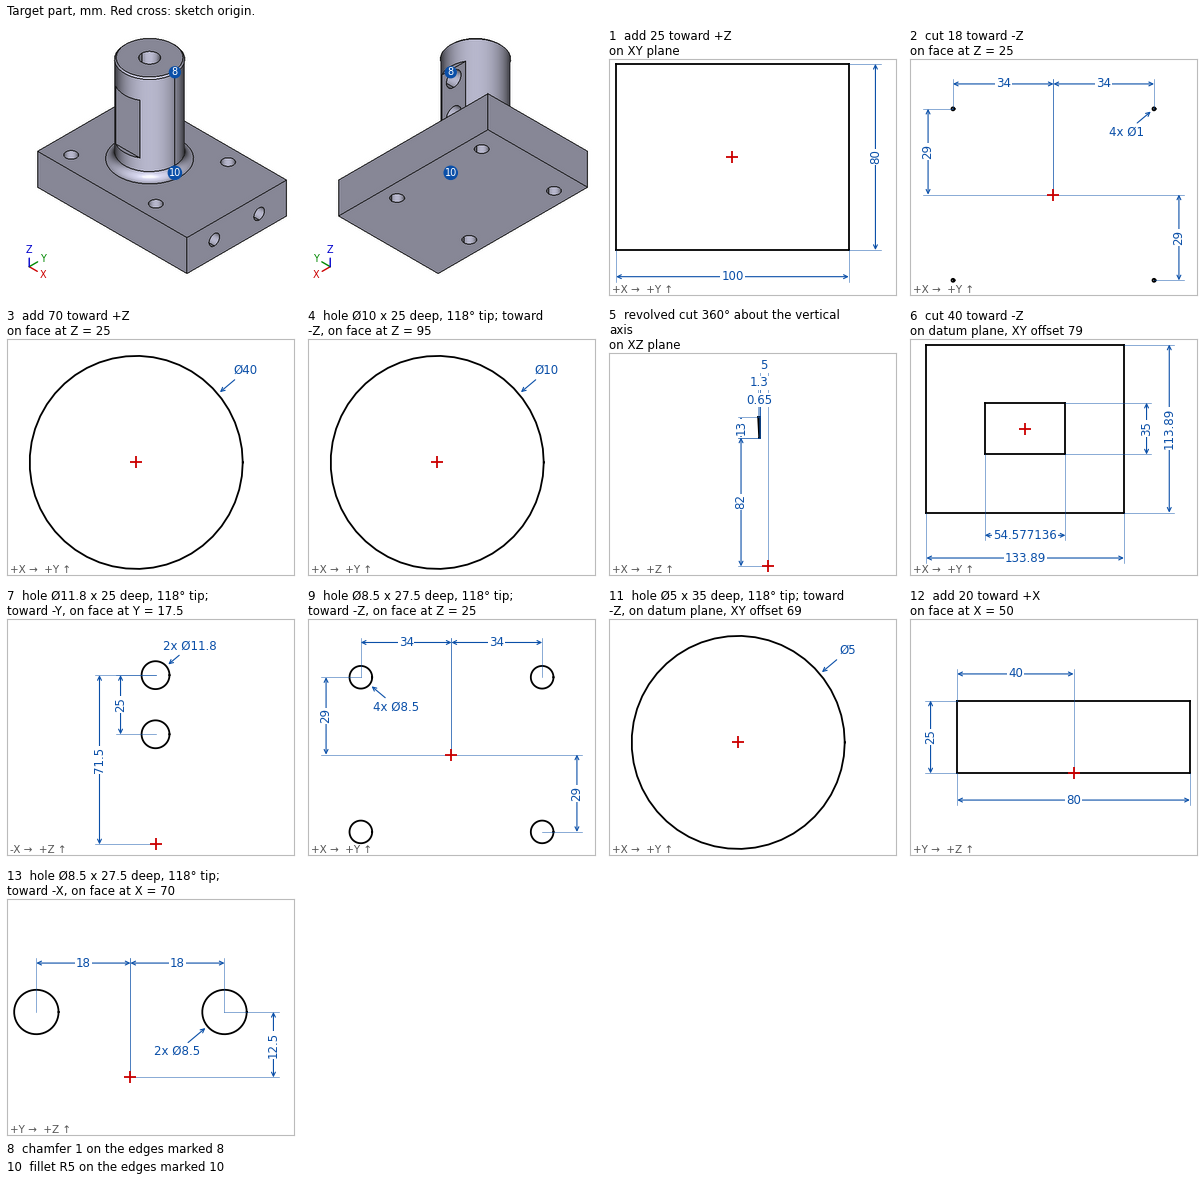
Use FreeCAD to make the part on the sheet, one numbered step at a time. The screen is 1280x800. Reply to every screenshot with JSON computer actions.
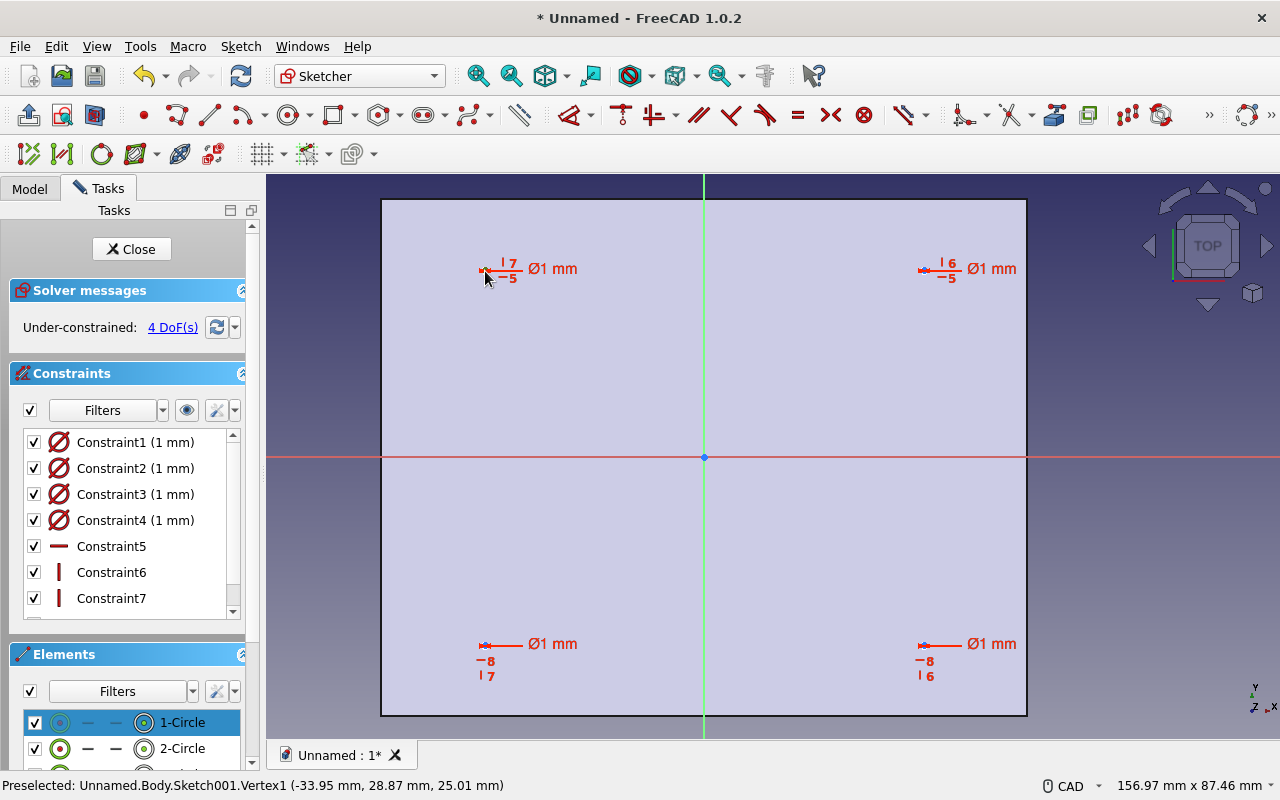
{"action": "key", "text": "l"}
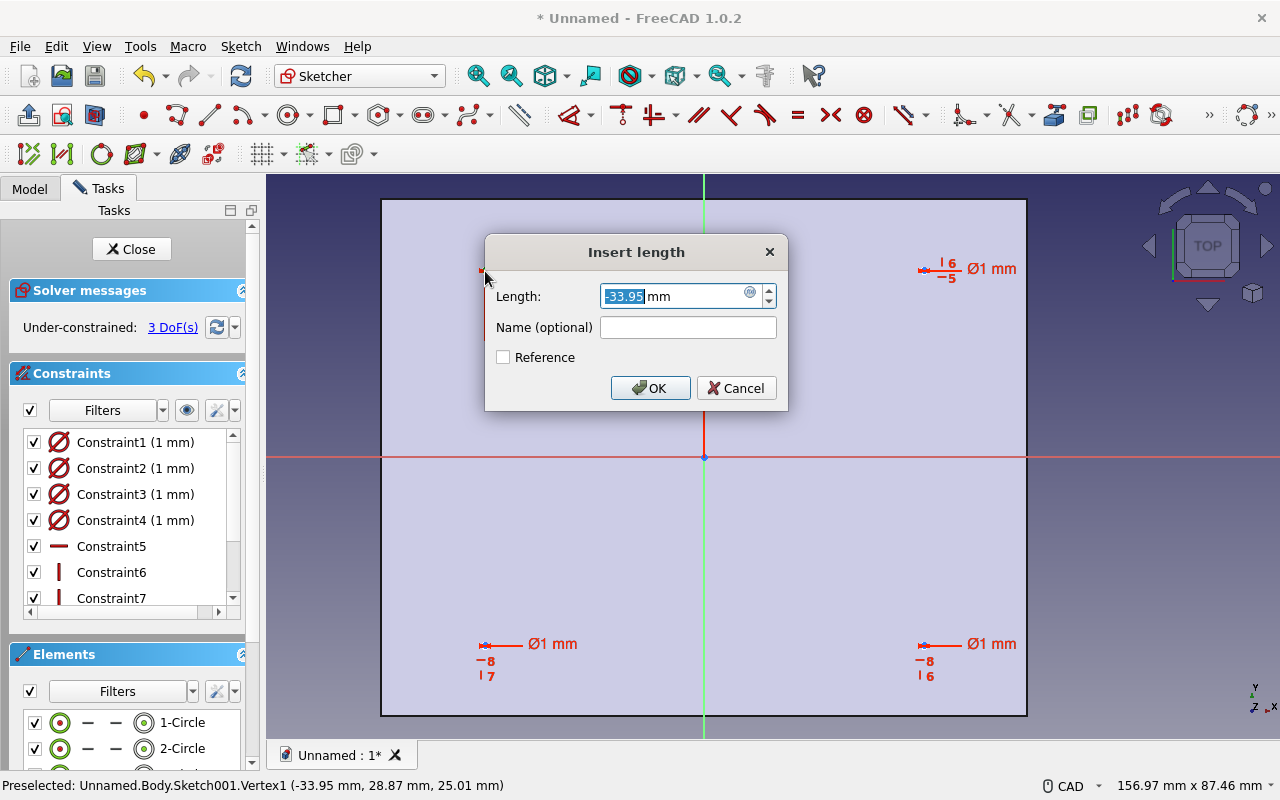
{"action": "type", "text": "-34"}
{"action": "key", "text": "Return"}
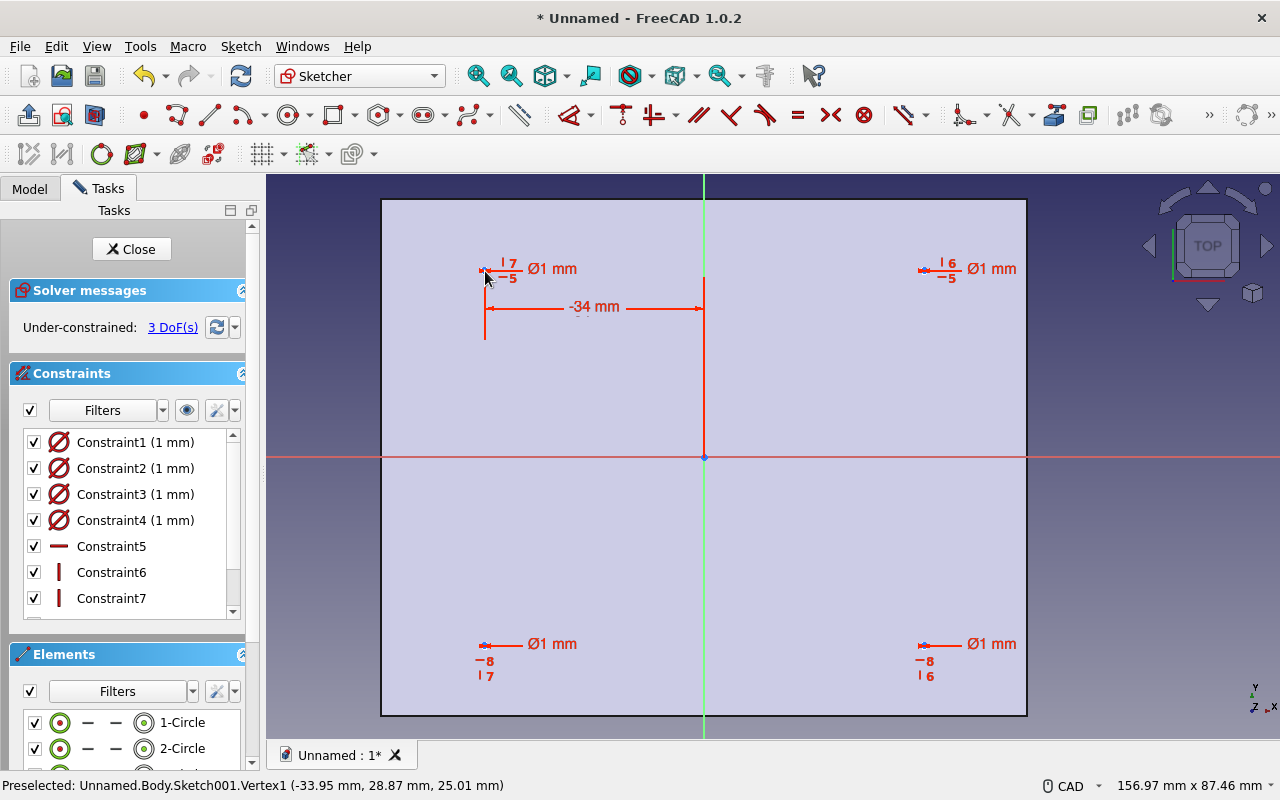
{"action": "left_click", "coordinate": [485, 271]}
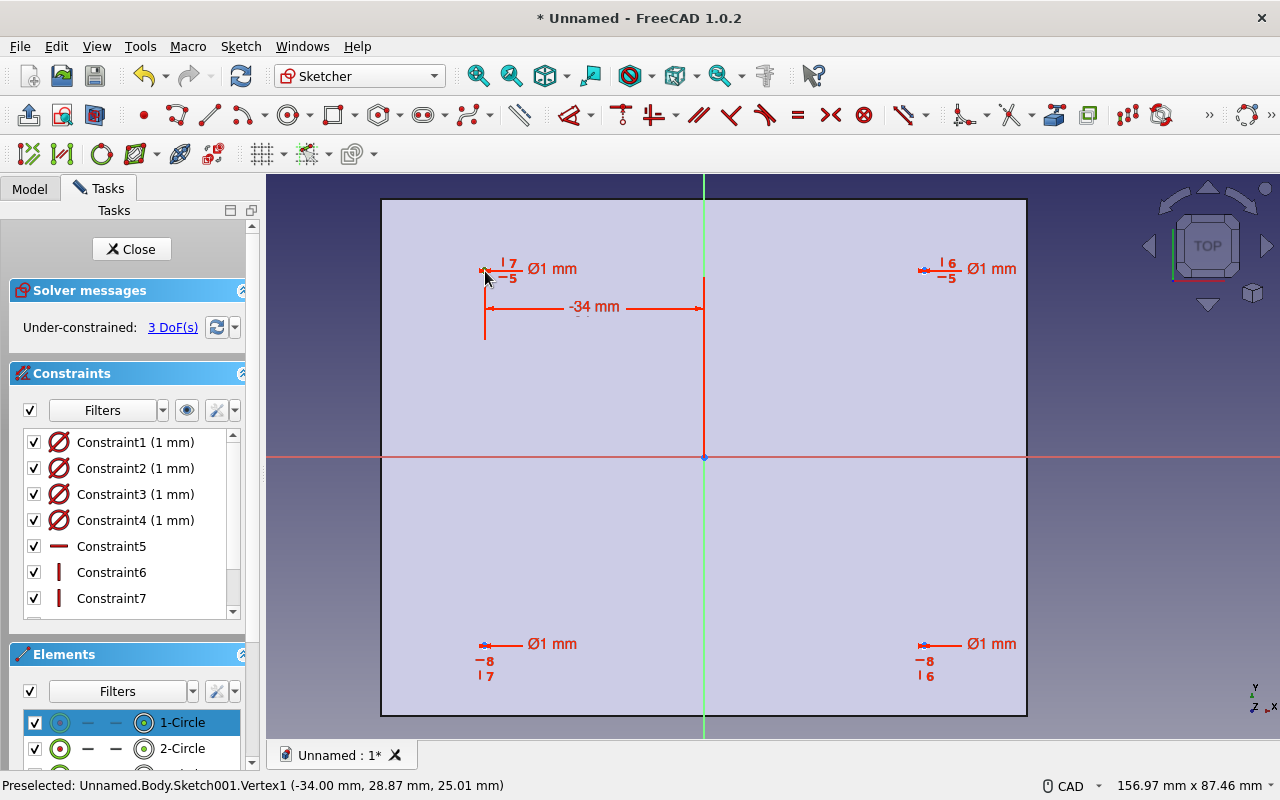
{"action": "key", "text": "i"}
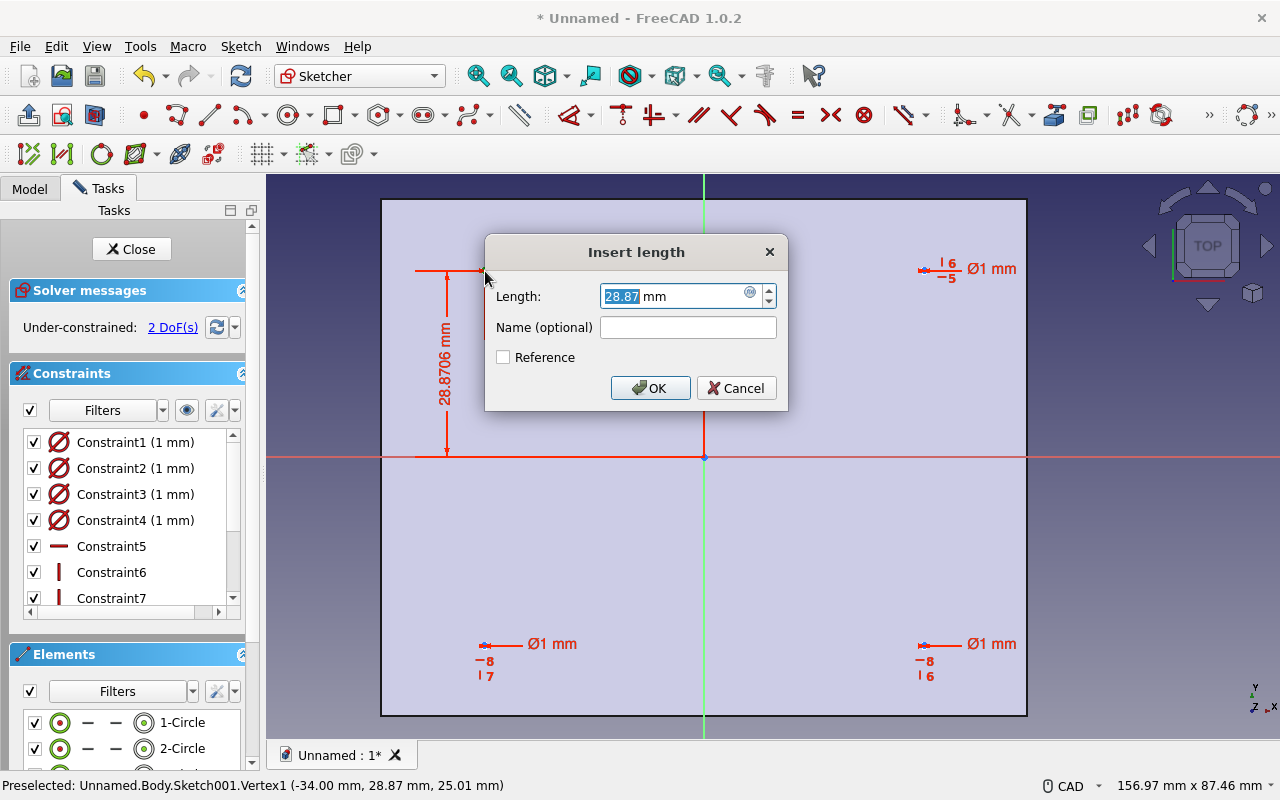
{"action": "type", "text": "29"}
{"action": "key", "text": "Return"}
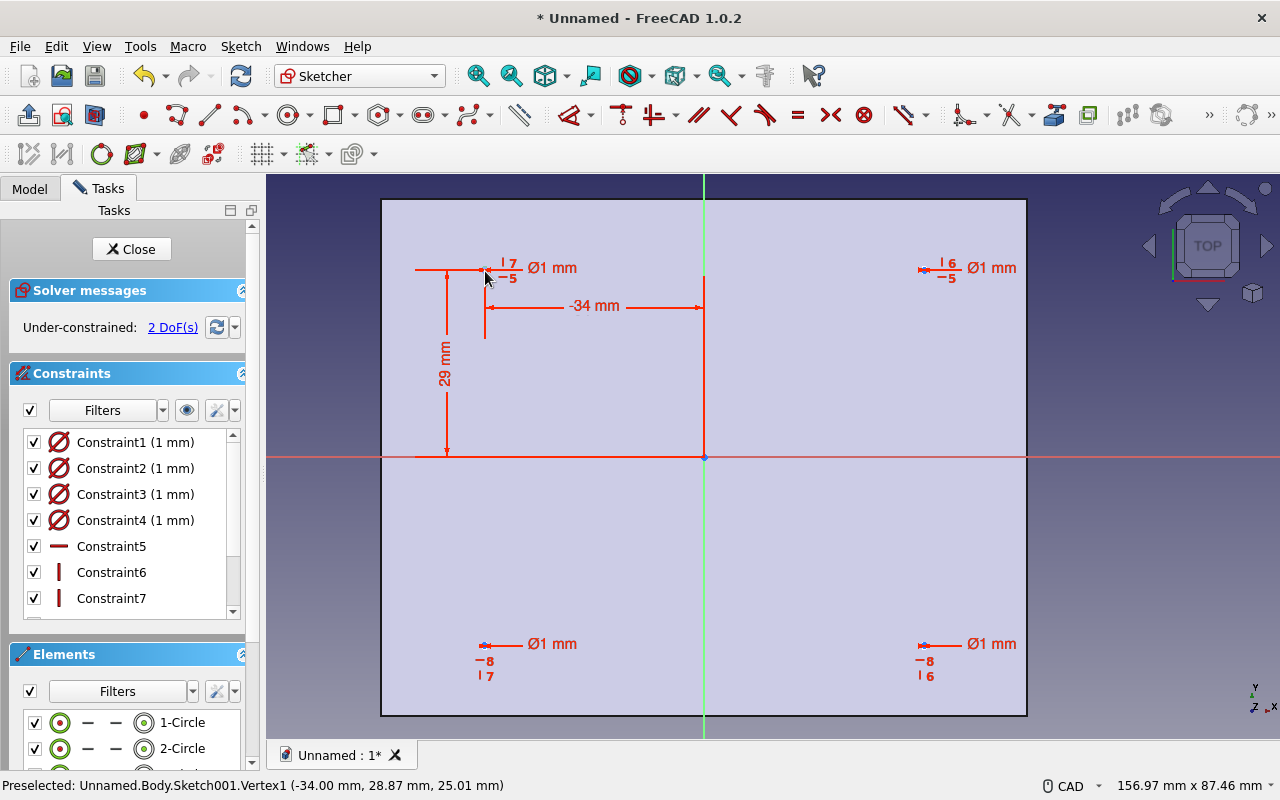
{"action": "left_click", "coordinate": [924, 270]}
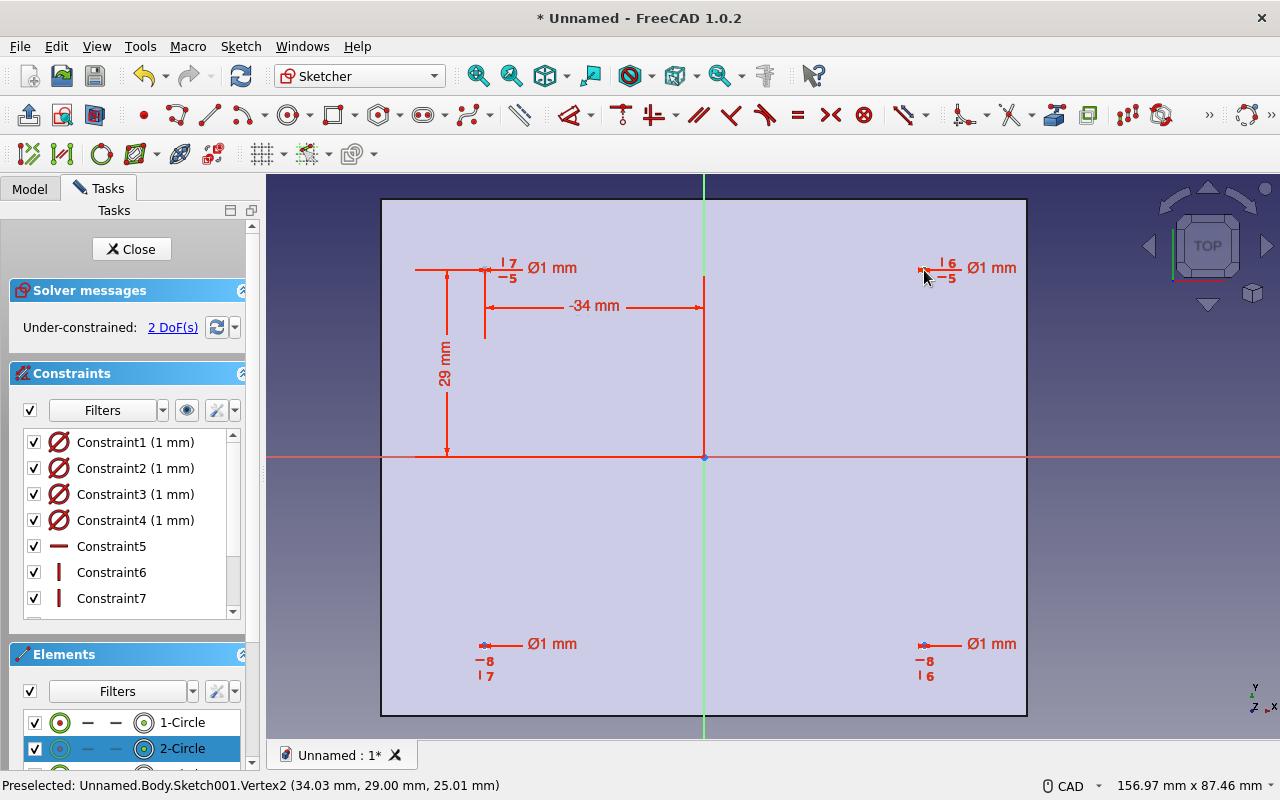
{"action": "key", "text": "l"}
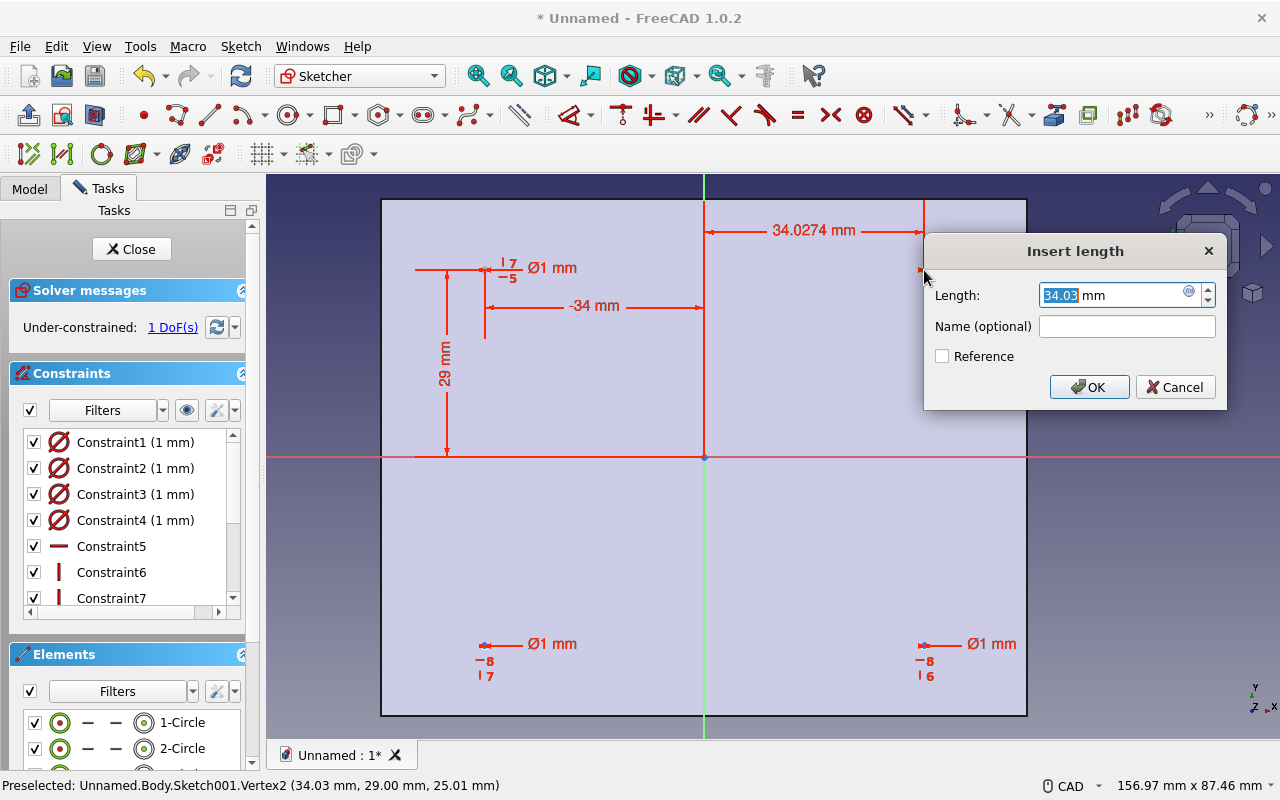
{"action": "type", "text": "34"}
{"action": "key", "text": "Return"}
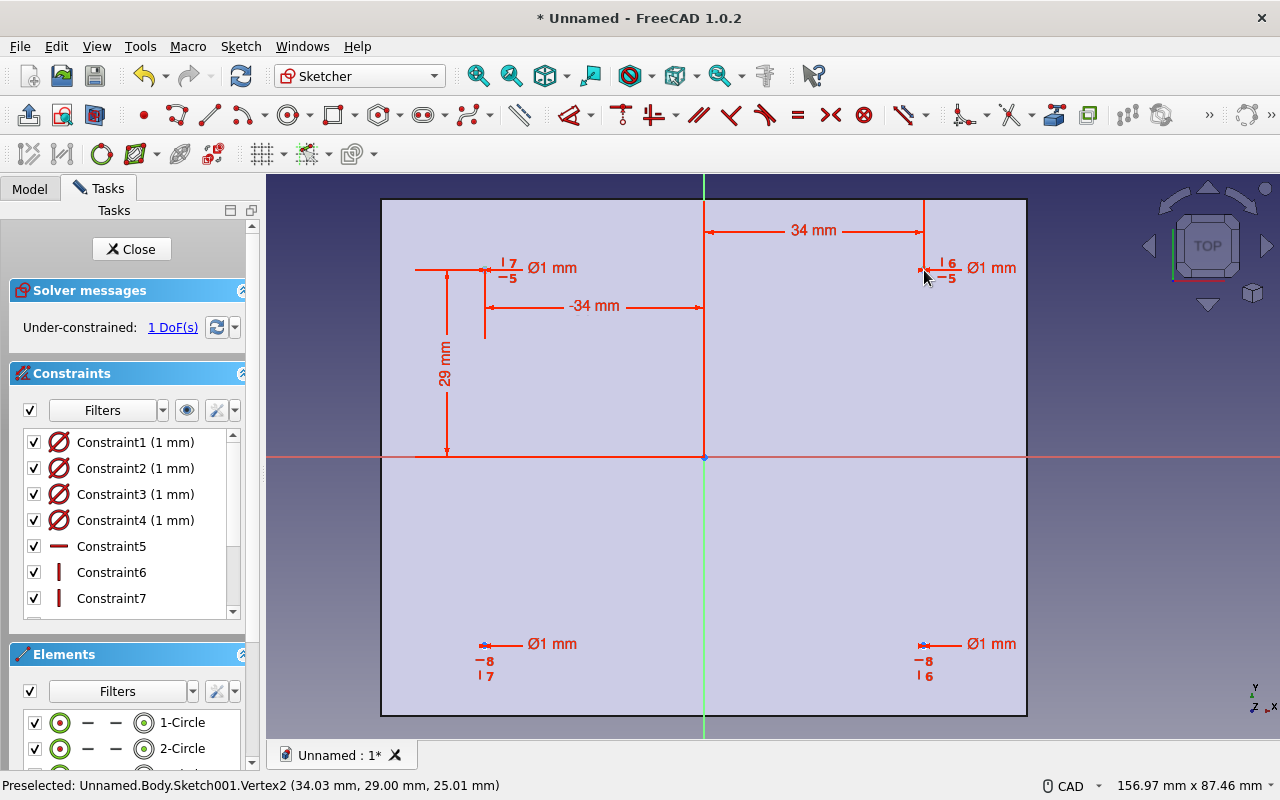
{"action": "left_click", "coordinate": [924, 646]}